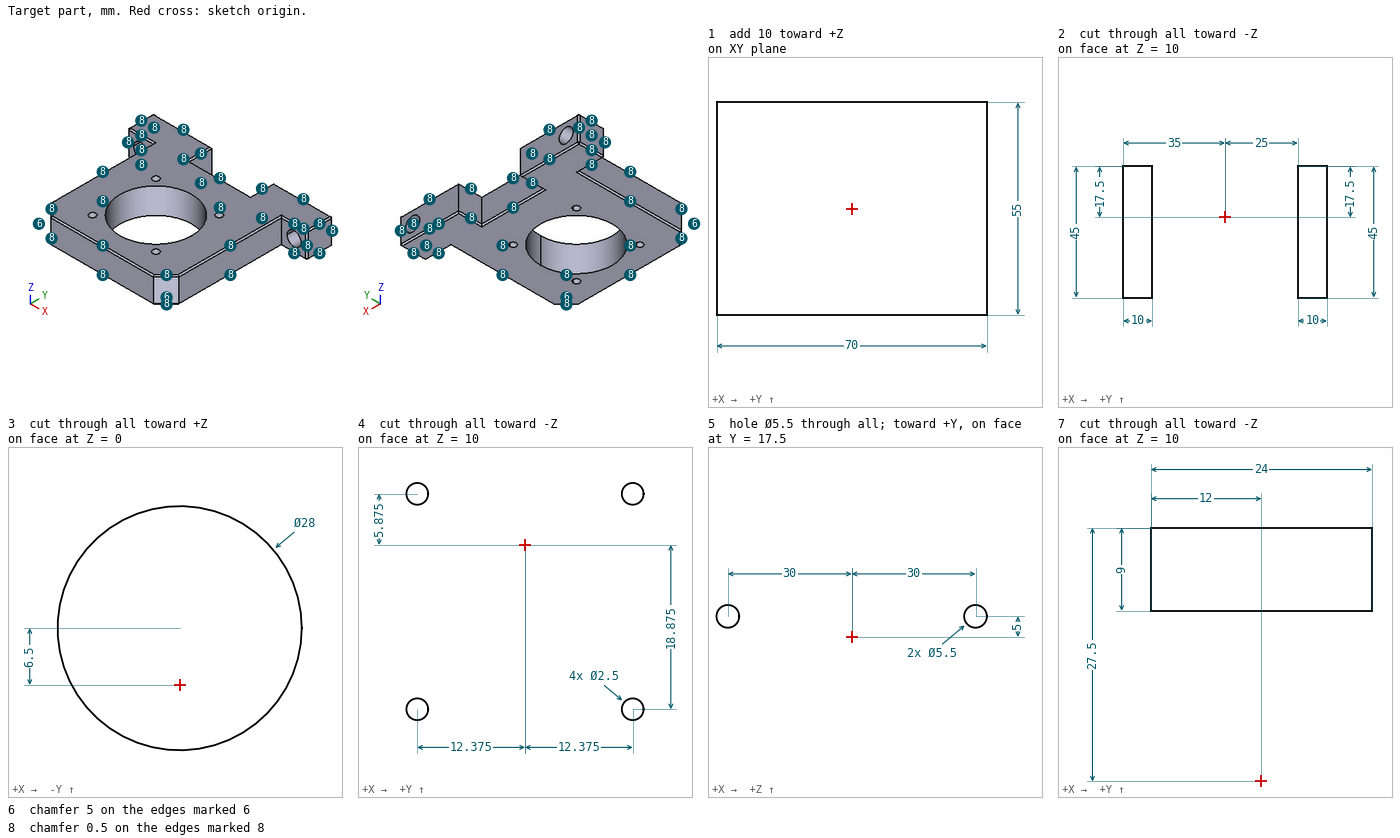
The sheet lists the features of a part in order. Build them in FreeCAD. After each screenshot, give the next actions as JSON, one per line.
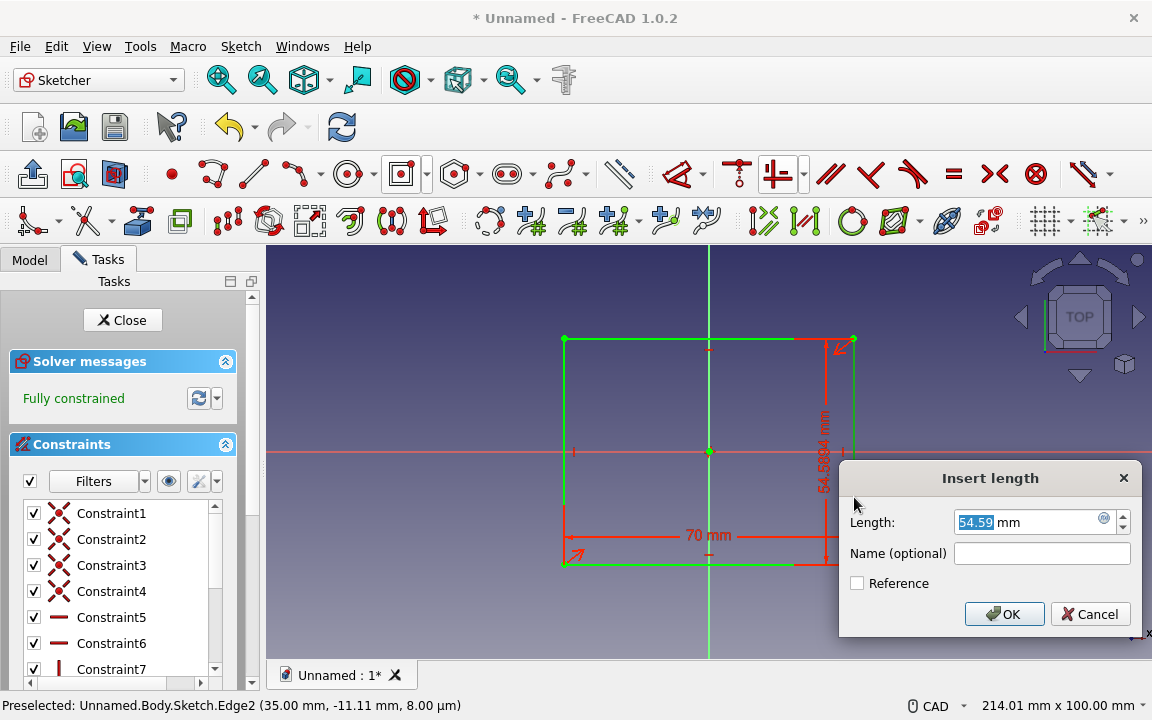
{"action": "type", "text": "55"}
{"action": "key", "text": "Return"}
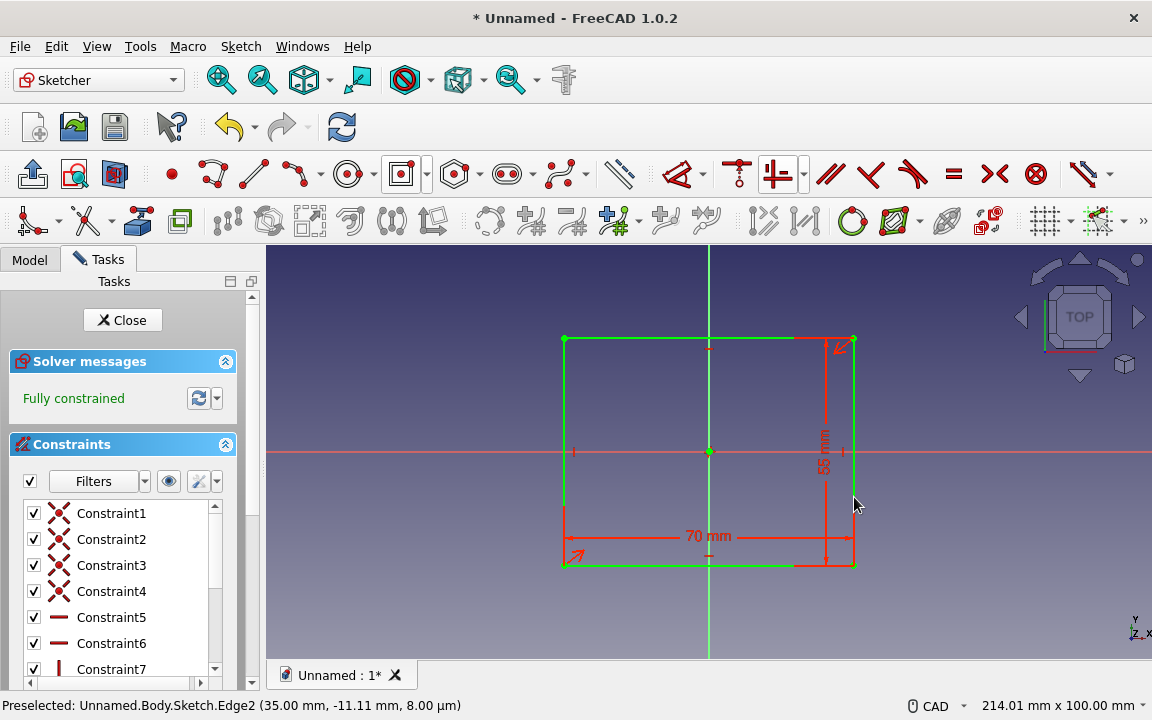
{"action": "left_click", "coordinate": [123, 320]}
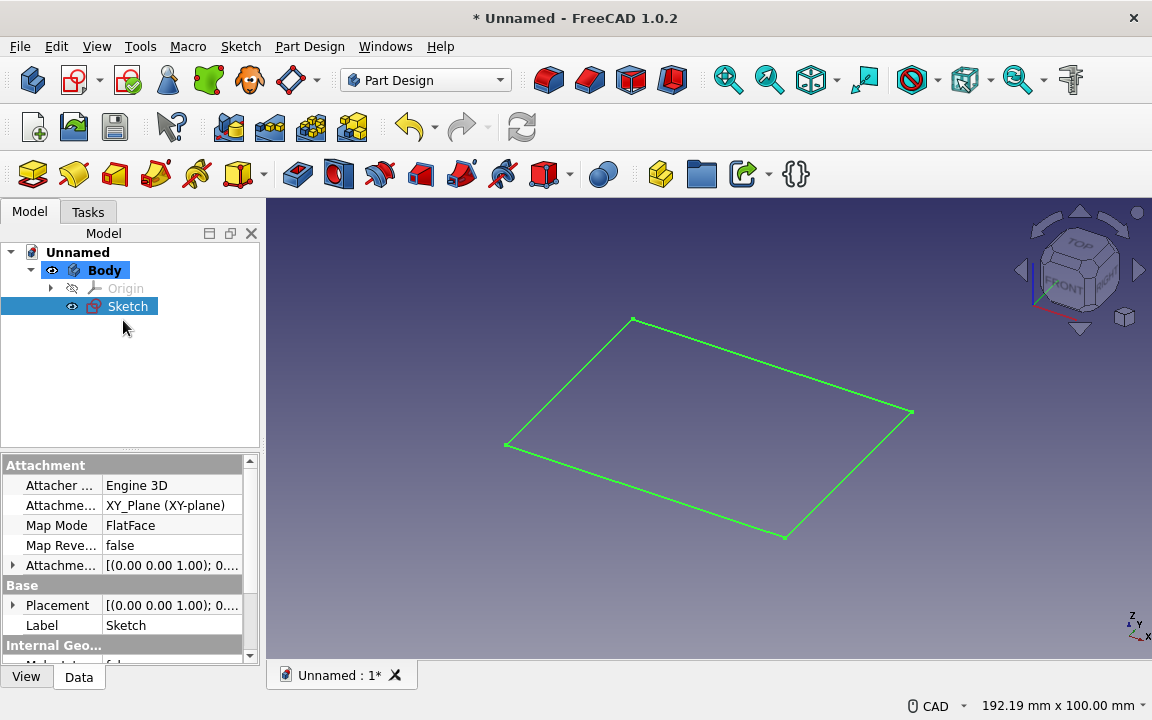
{"action": "left_click", "coordinate": [33, 174]}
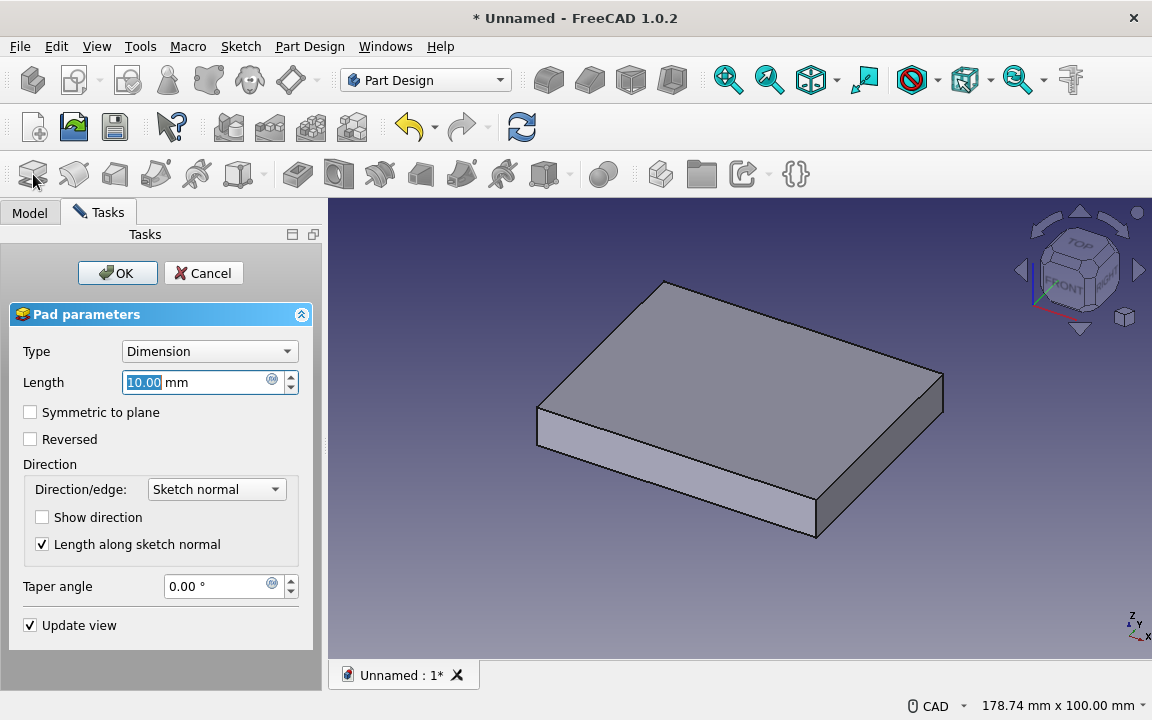
{"action": "type", "text": "10"}
{"action": "key", "text": "Tab"}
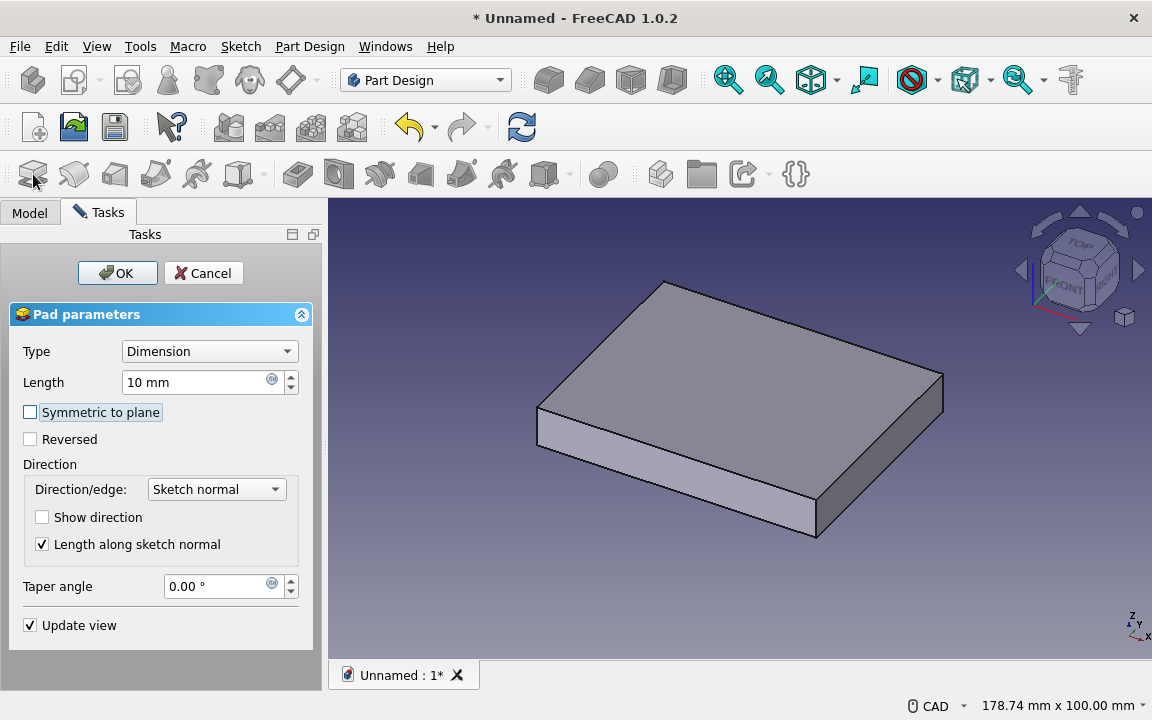
{"action": "left_click", "coordinate": [118, 273]}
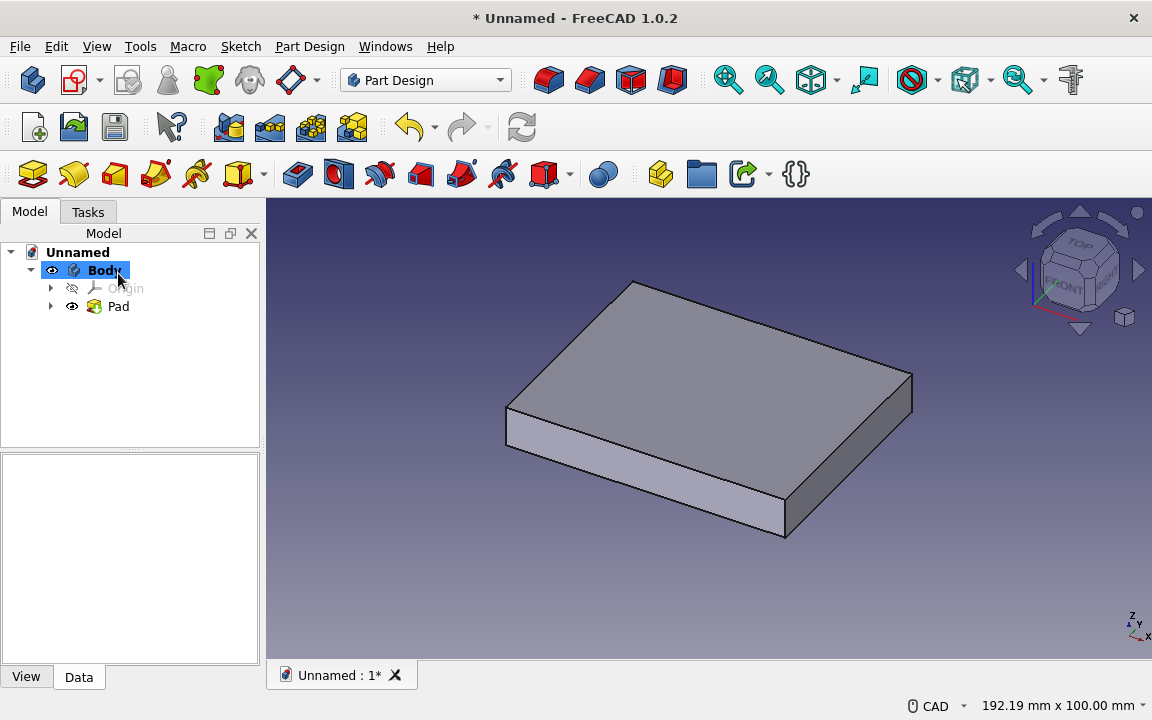
{"action": "left_click", "coordinate": [709, 390]}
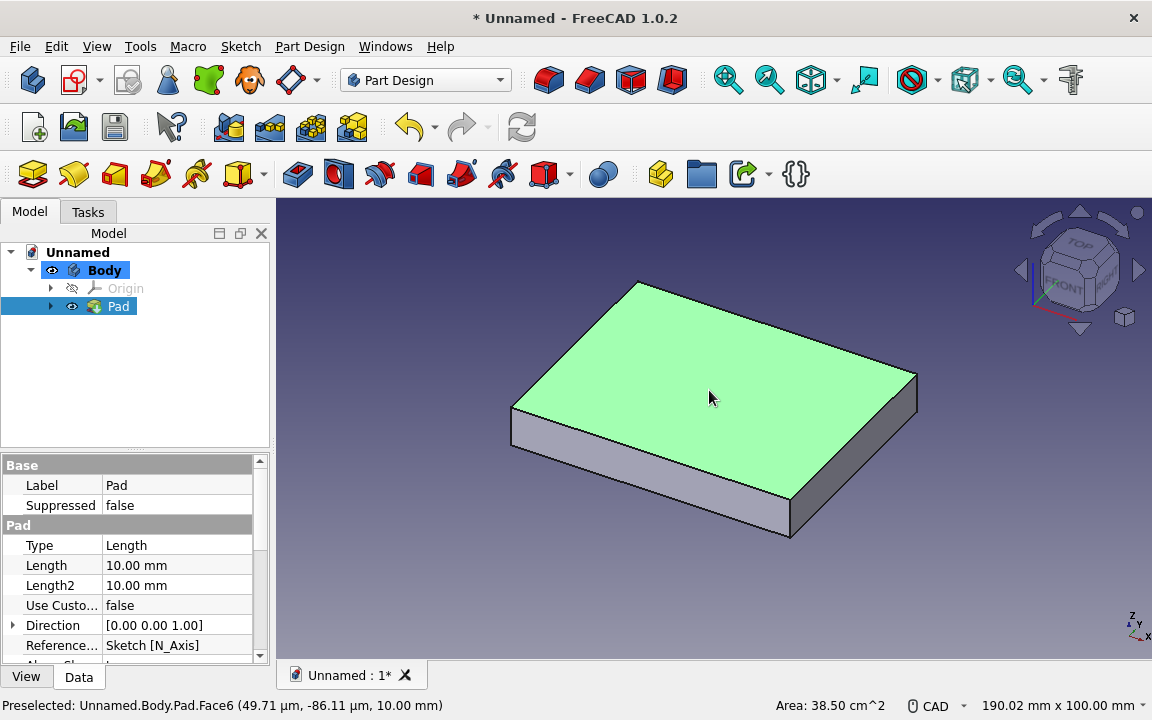
{"action": "left_click", "coordinate": [74, 80]}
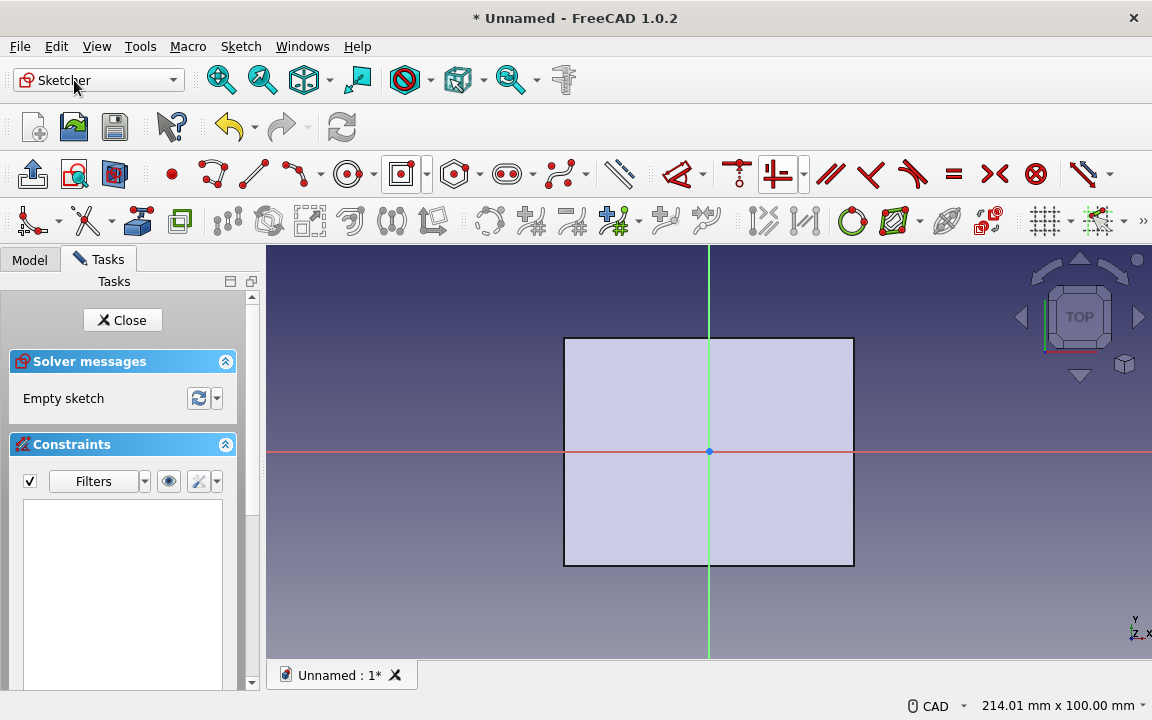
{"action": "scroll", "coordinate": [848, 515], "scroll_direction": "up", "scroll_amount": 2}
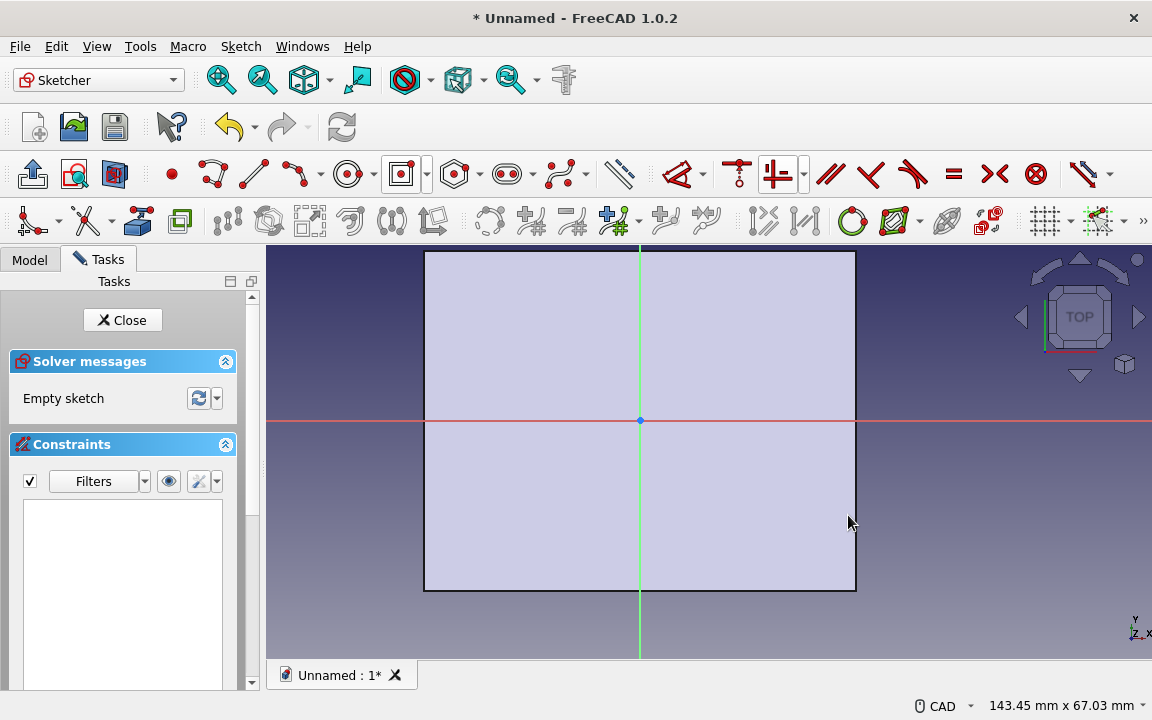
{"action": "left_click", "coordinate": [426, 174]}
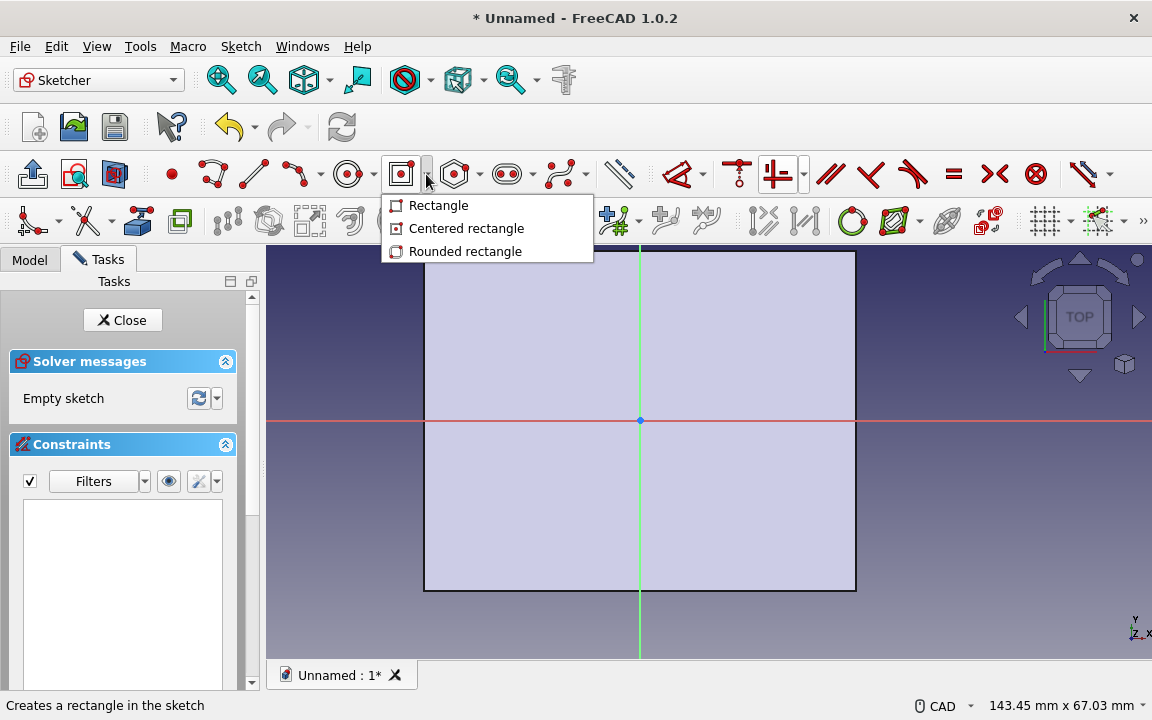
{"action": "left_click", "coordinate": [488, 206]}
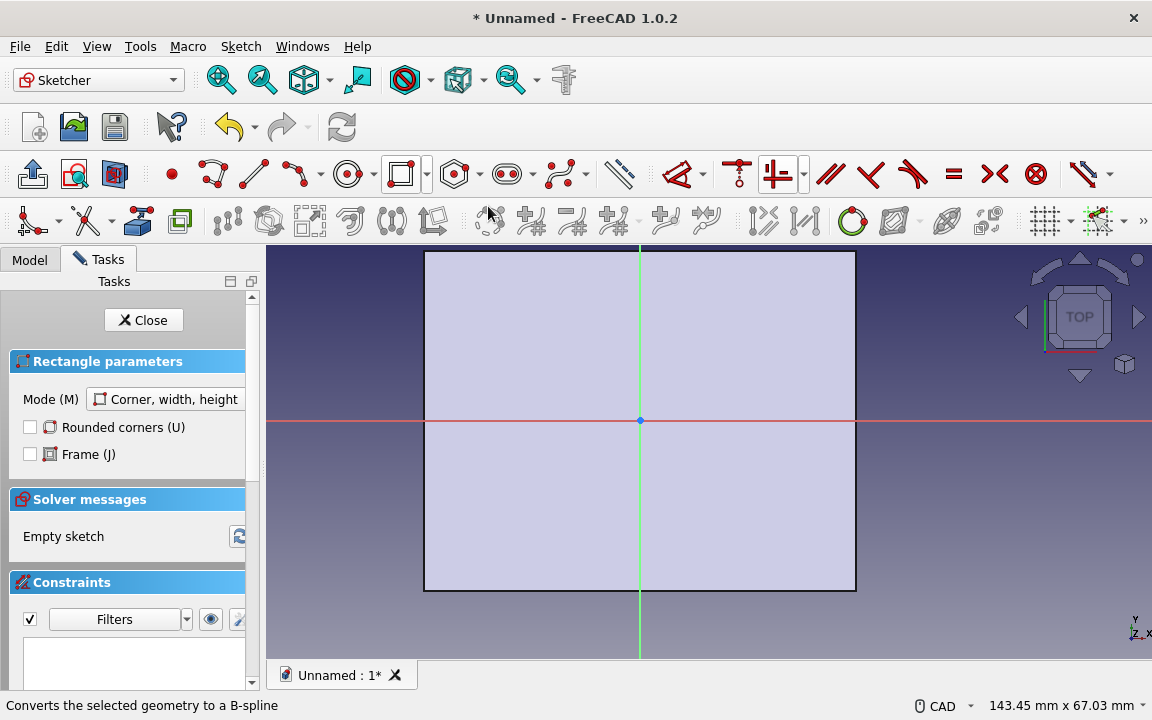
{"action": "left_click", "coordinate": [424, 313]}
{"action": "left_click", "coordinate": [486, 591]}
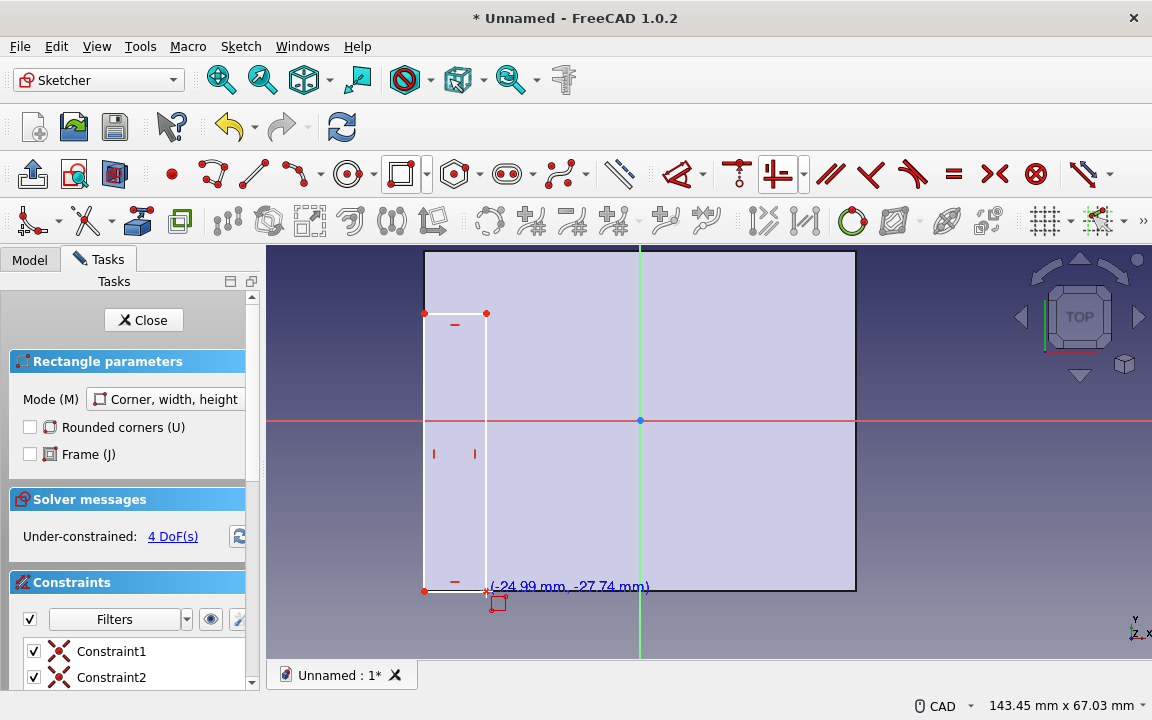
{"action": "left_click", "coordinate": [795, 313]}
{"action": "left_click", "coordinate": [856, 591]}
{"action": "key", "text": "Escape"}